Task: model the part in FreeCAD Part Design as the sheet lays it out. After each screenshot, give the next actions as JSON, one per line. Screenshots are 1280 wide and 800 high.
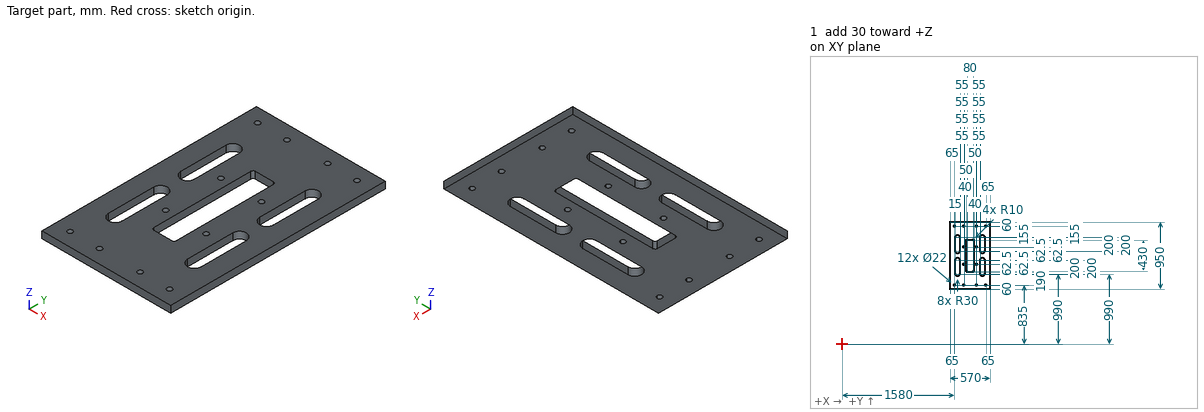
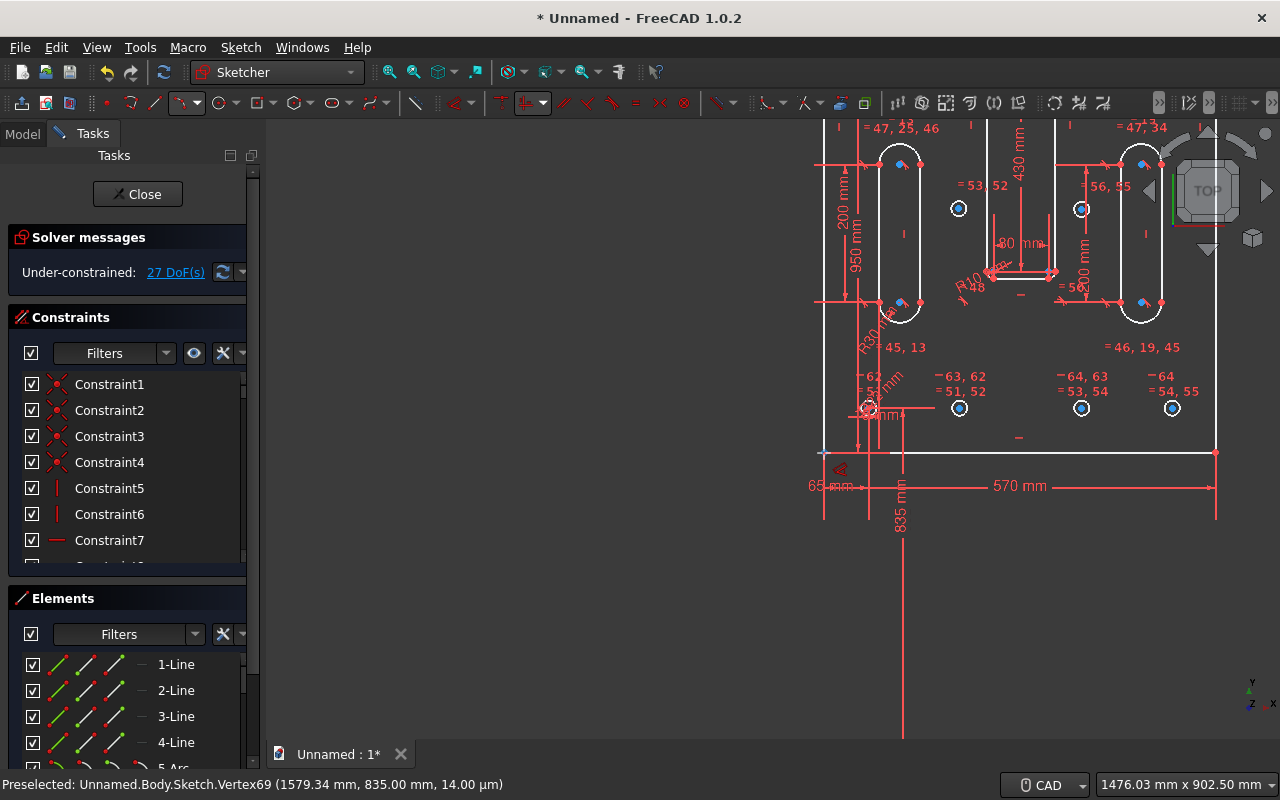
{"action": "left_click", "coordinate": [824, 453]}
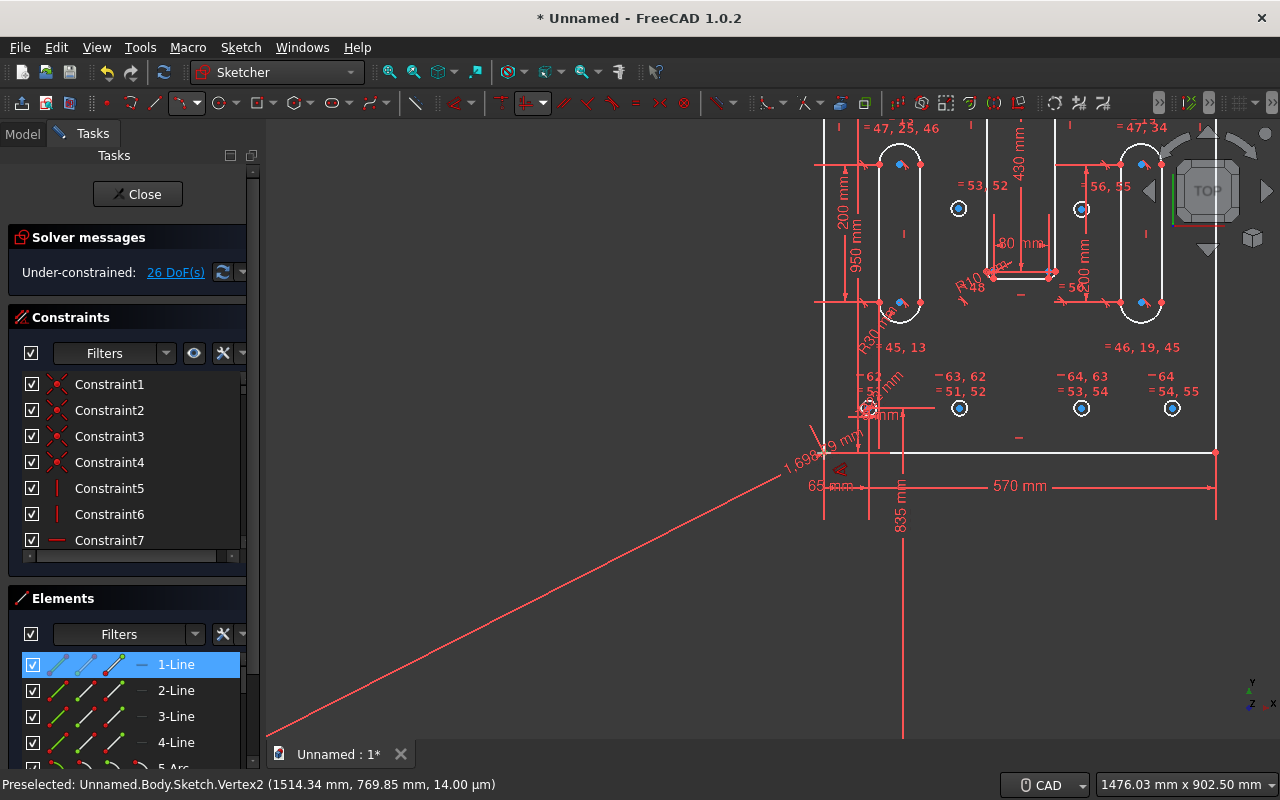
{"action": "left_click", "coordinate": [869, 408]}
{"action": "left_click", "coordinate": [790, 430]}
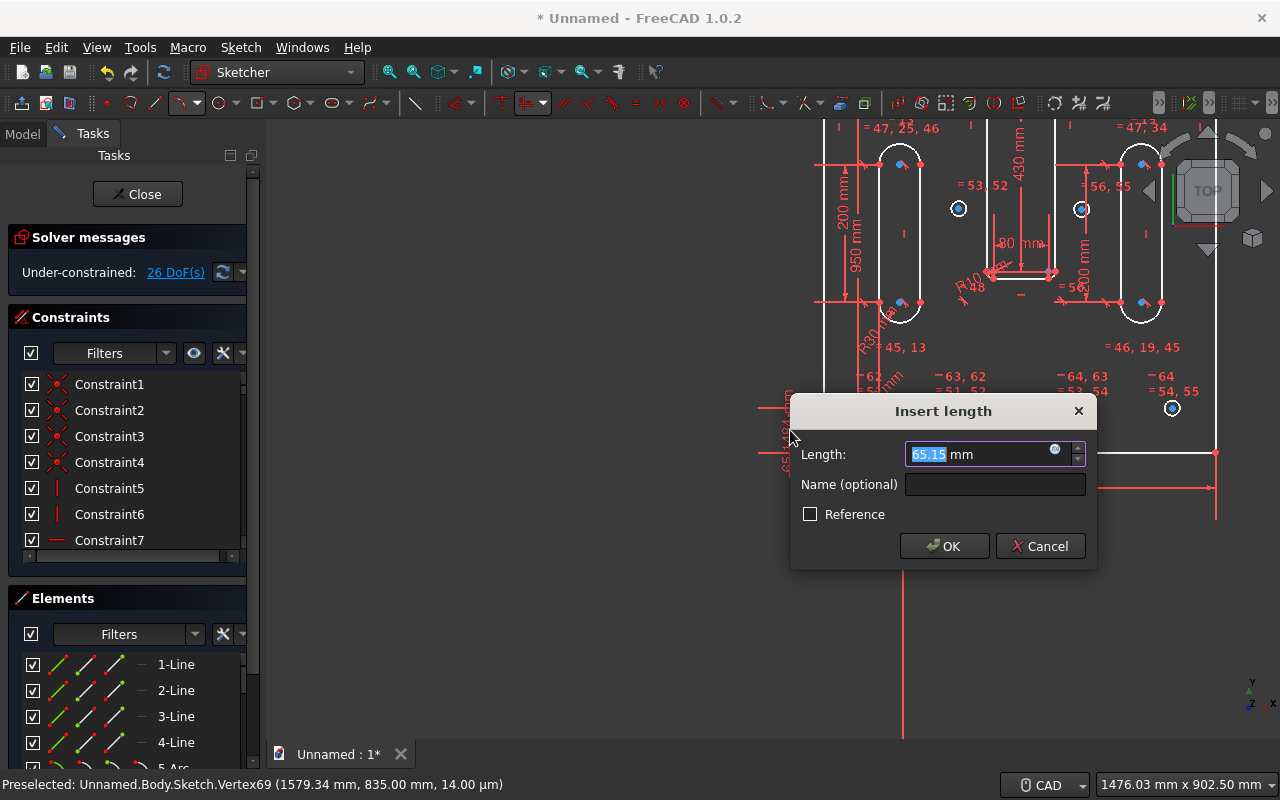
{"action": "type", "text": "60"}
{"action": "key", "text": "Return"}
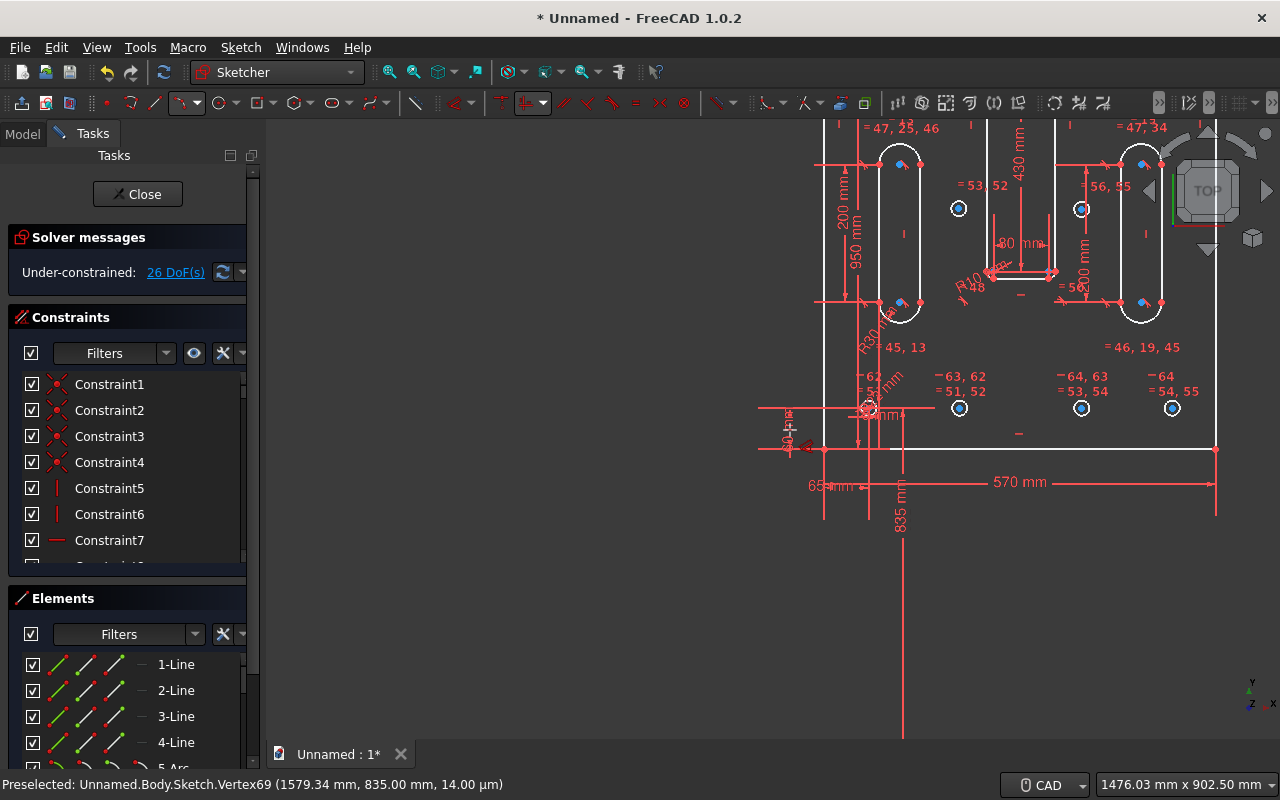
{"action": "left_click", "coordinate": [920, 302]}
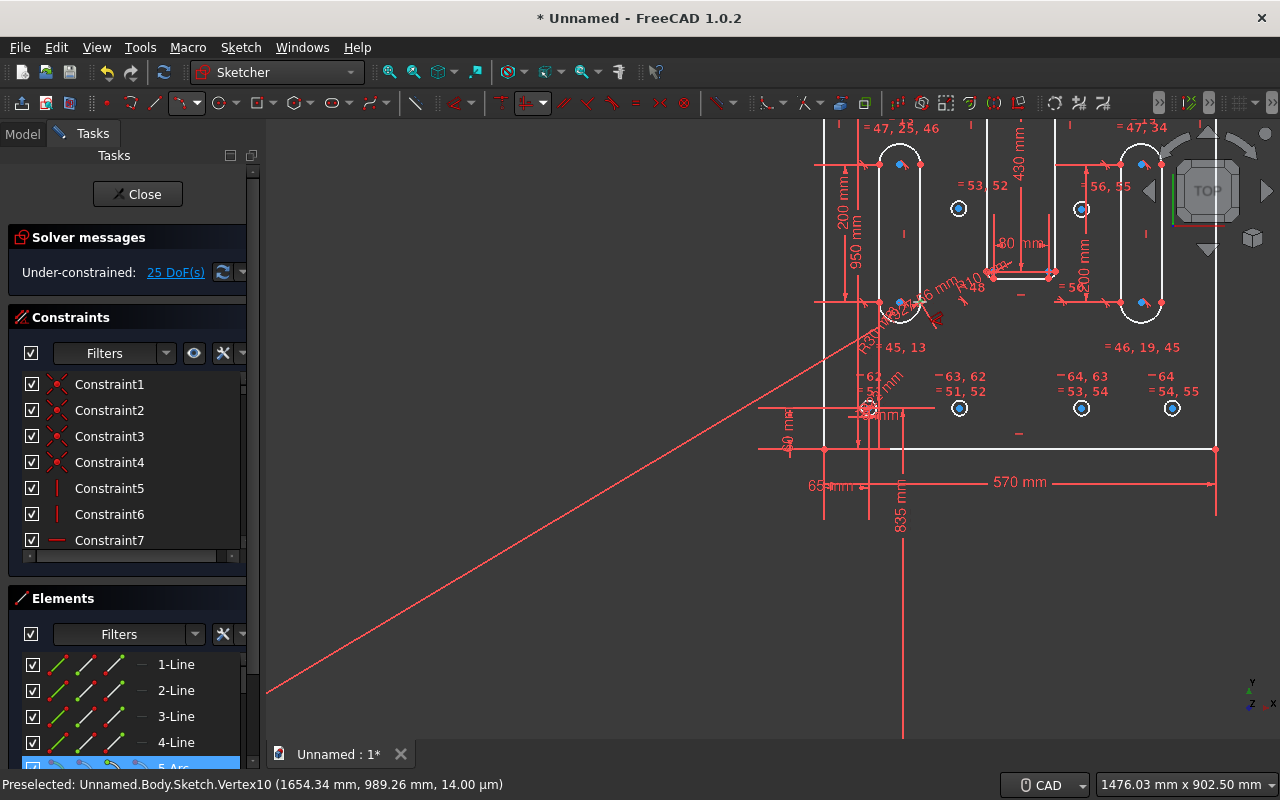
{"action": "left_click", "coordinate": [960, 408]}
{"action": "left_click", "coordinate": [940, 244]}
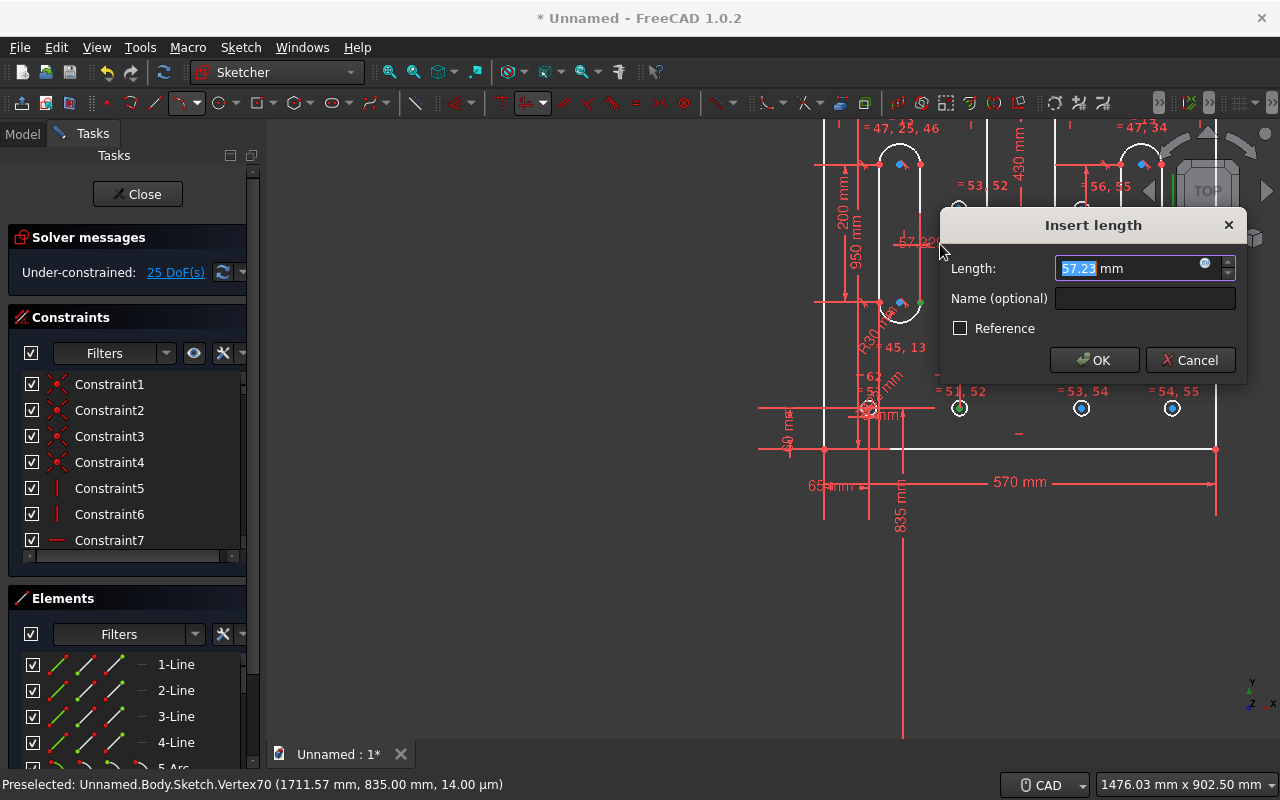
{"action": "type", "text": "55"}
{"action": "key", "text": "Return"}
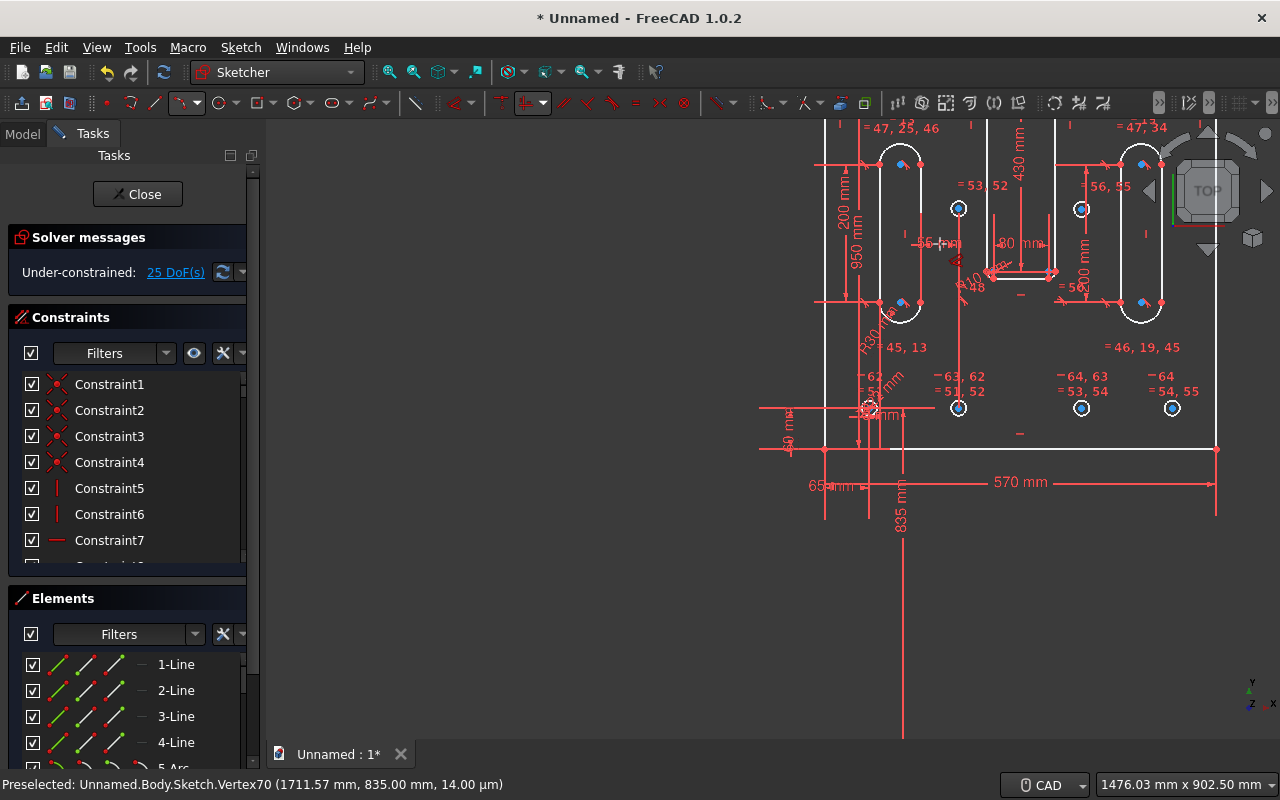
{"action": "scroll", "coordinate": [994, 279], "scroll_direction": "up", "scroll_amount": 3}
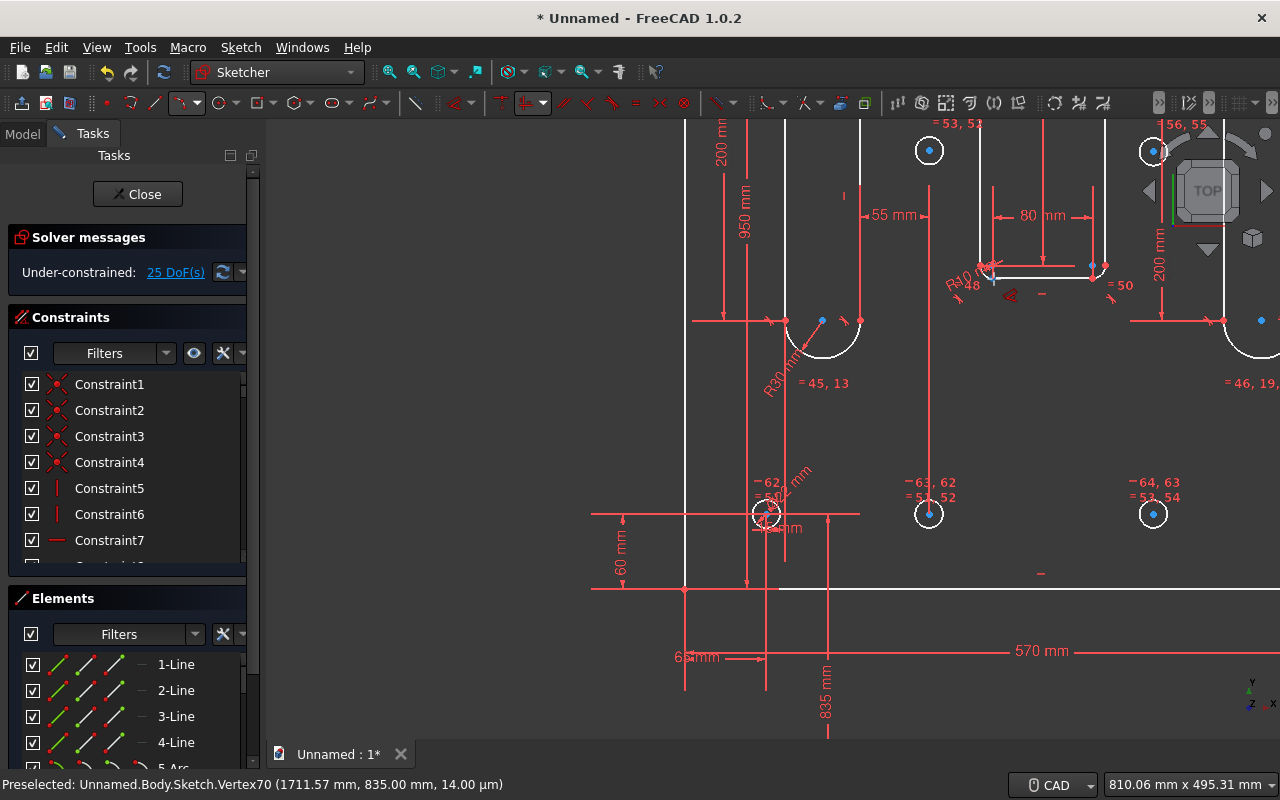
{"action": "left_click", "coordinate": [993, 278]}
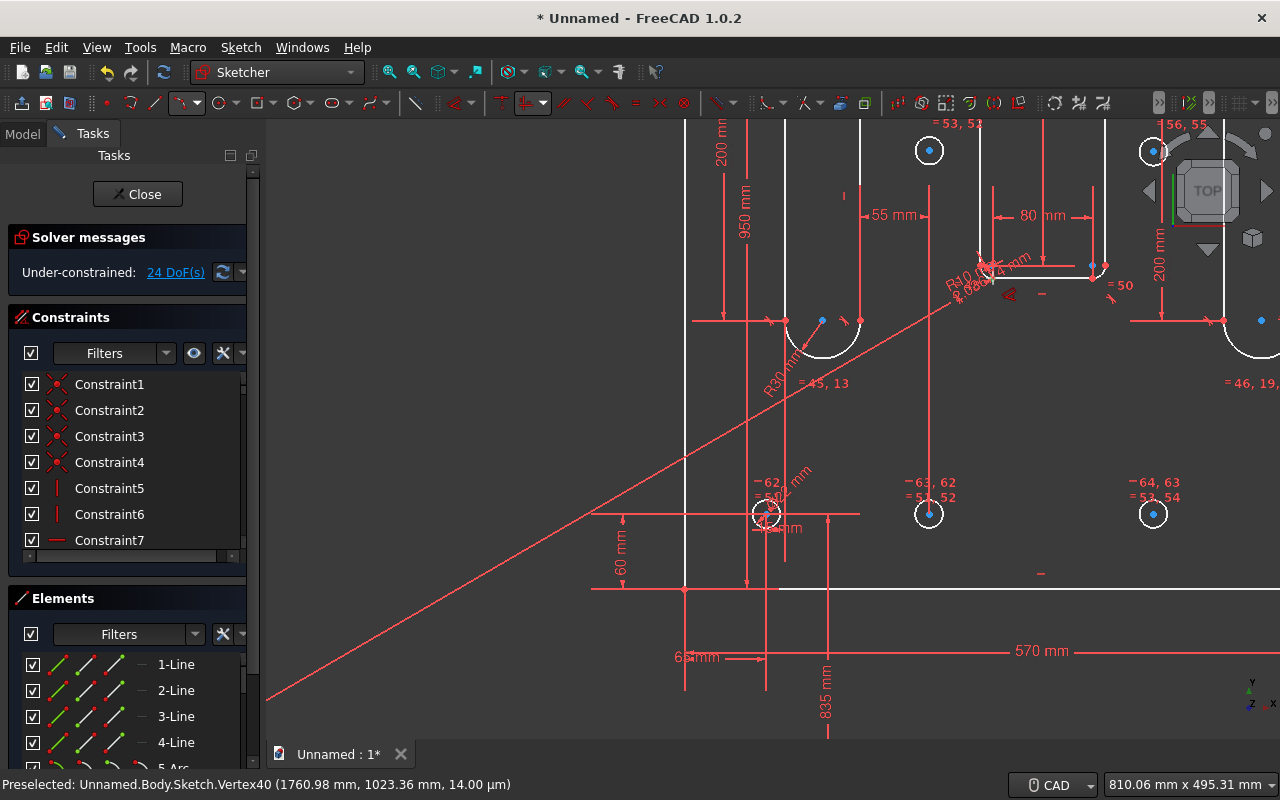
{"action": "left_click", "coordinate": [929, 514]}
{"action": "left_click", "coordinate": [961, 244]}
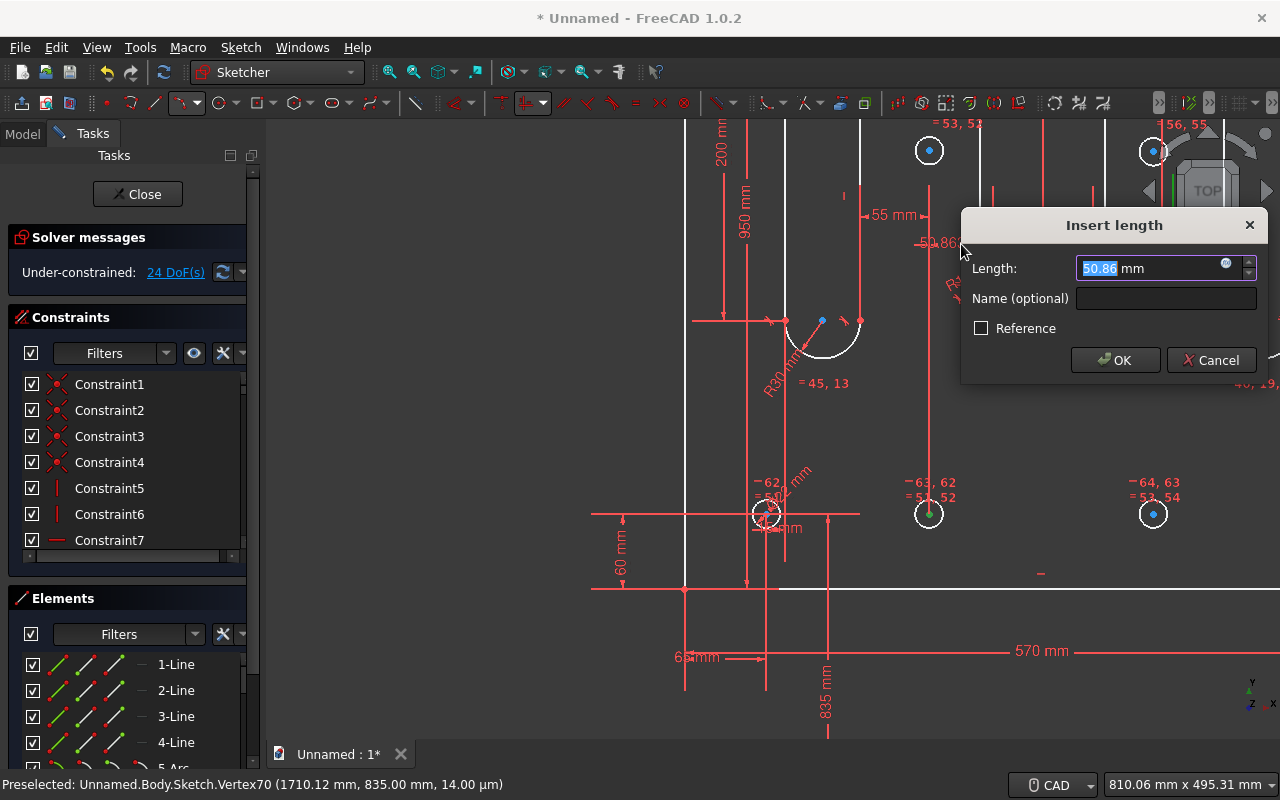
{"action": "type", "text": "50"}
{"action": "key", "text": "Return"}